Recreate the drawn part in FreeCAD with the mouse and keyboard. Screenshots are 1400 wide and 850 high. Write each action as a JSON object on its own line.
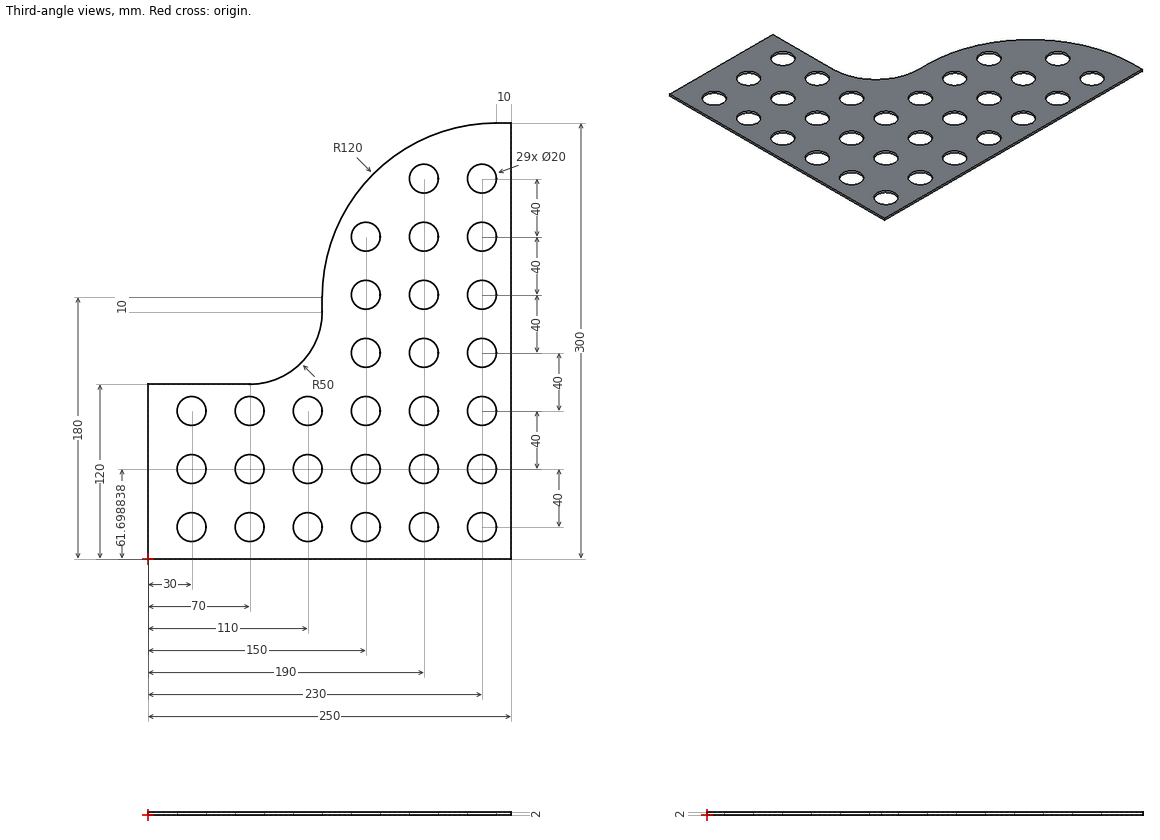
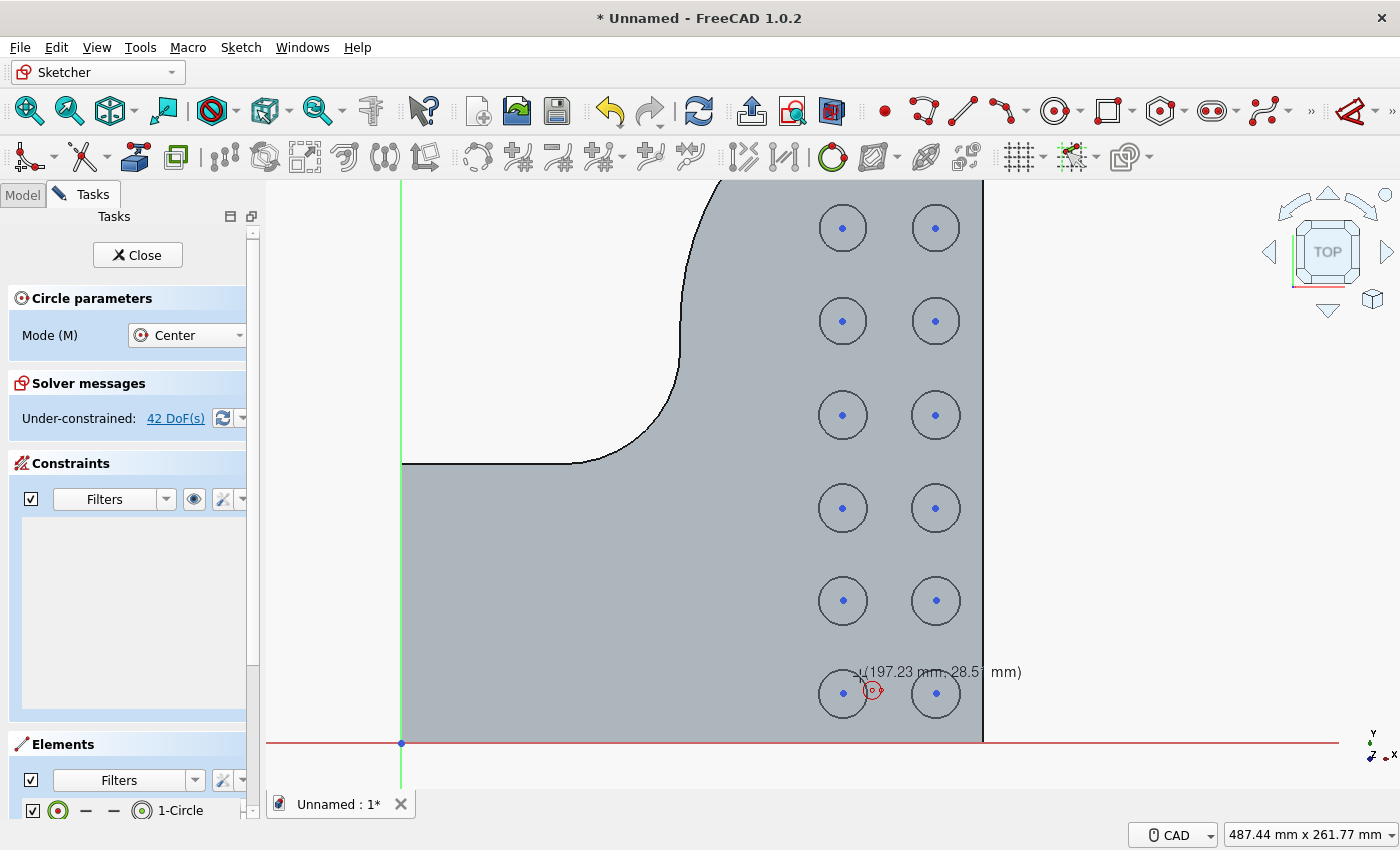
{"action": "left_click", "coordinate": [750, 228]}
{"action": "left_click", "coordinate": [767, 211]}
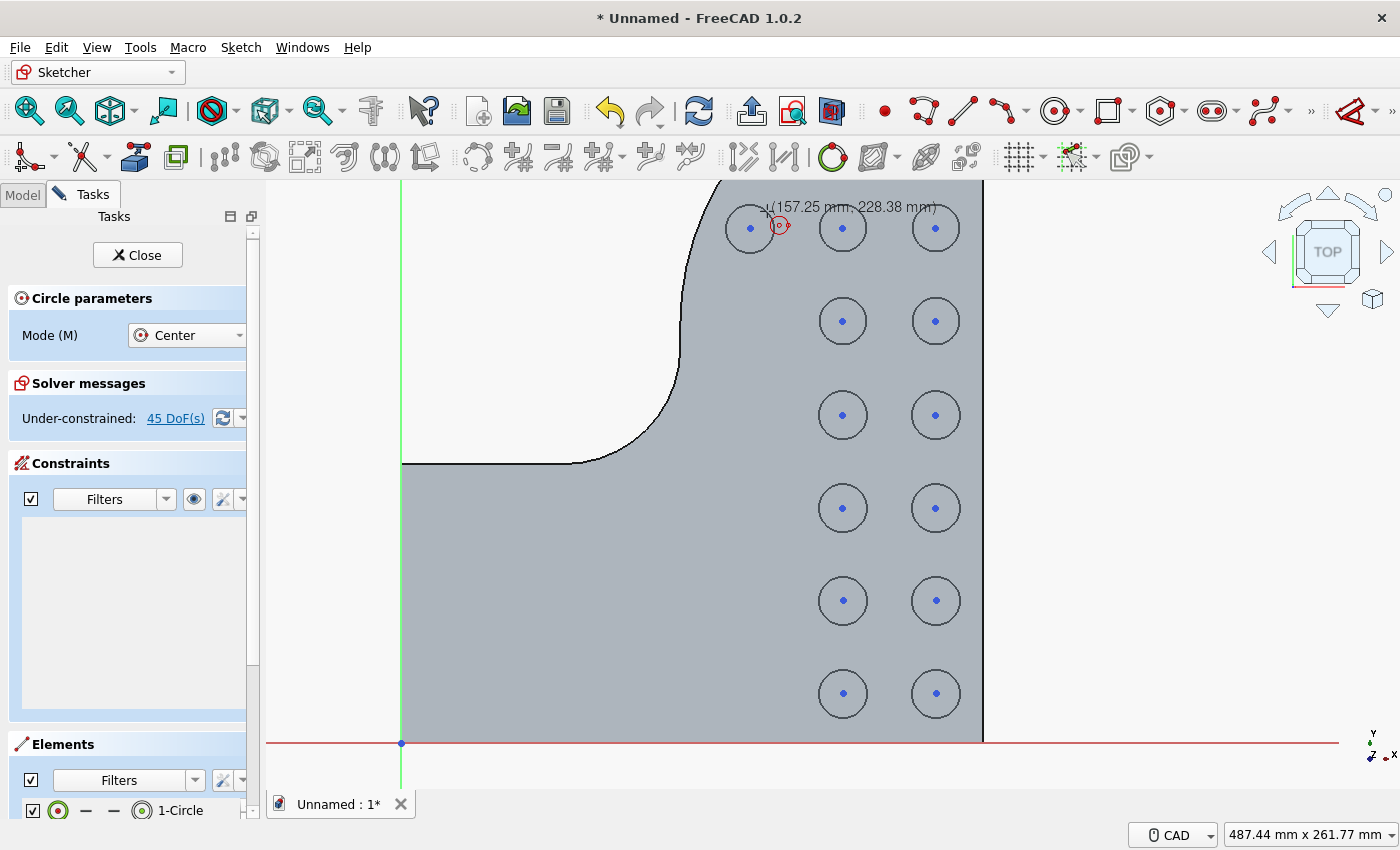
{"action": "left_click", "coordinate": [750, 321]}
{"action": "left_click", "coordinate": [767, 304]}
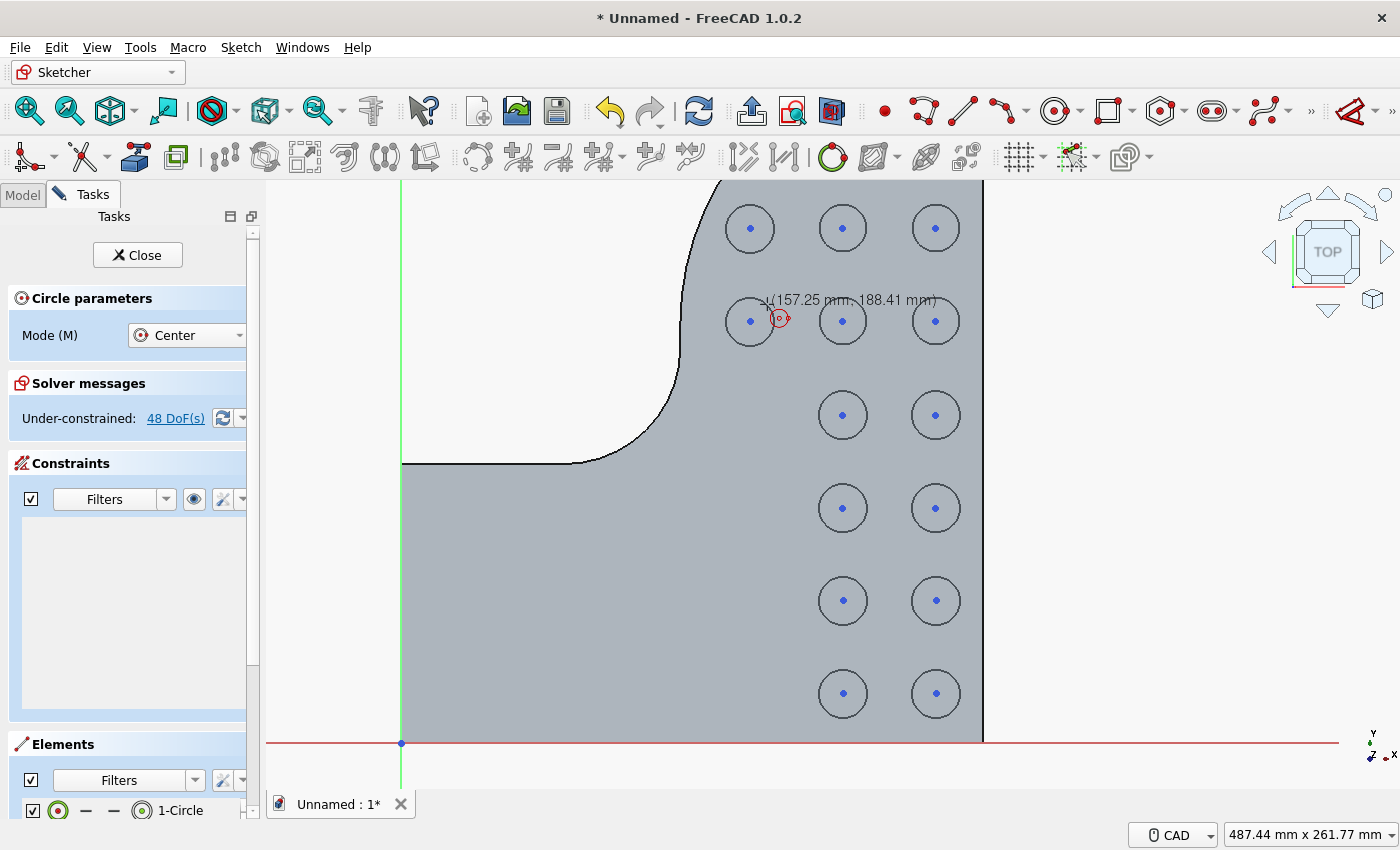
{"action": "left_click", "coordinate": [750, 414]}
{"action": "left_click", "coordinate": [767, 397]}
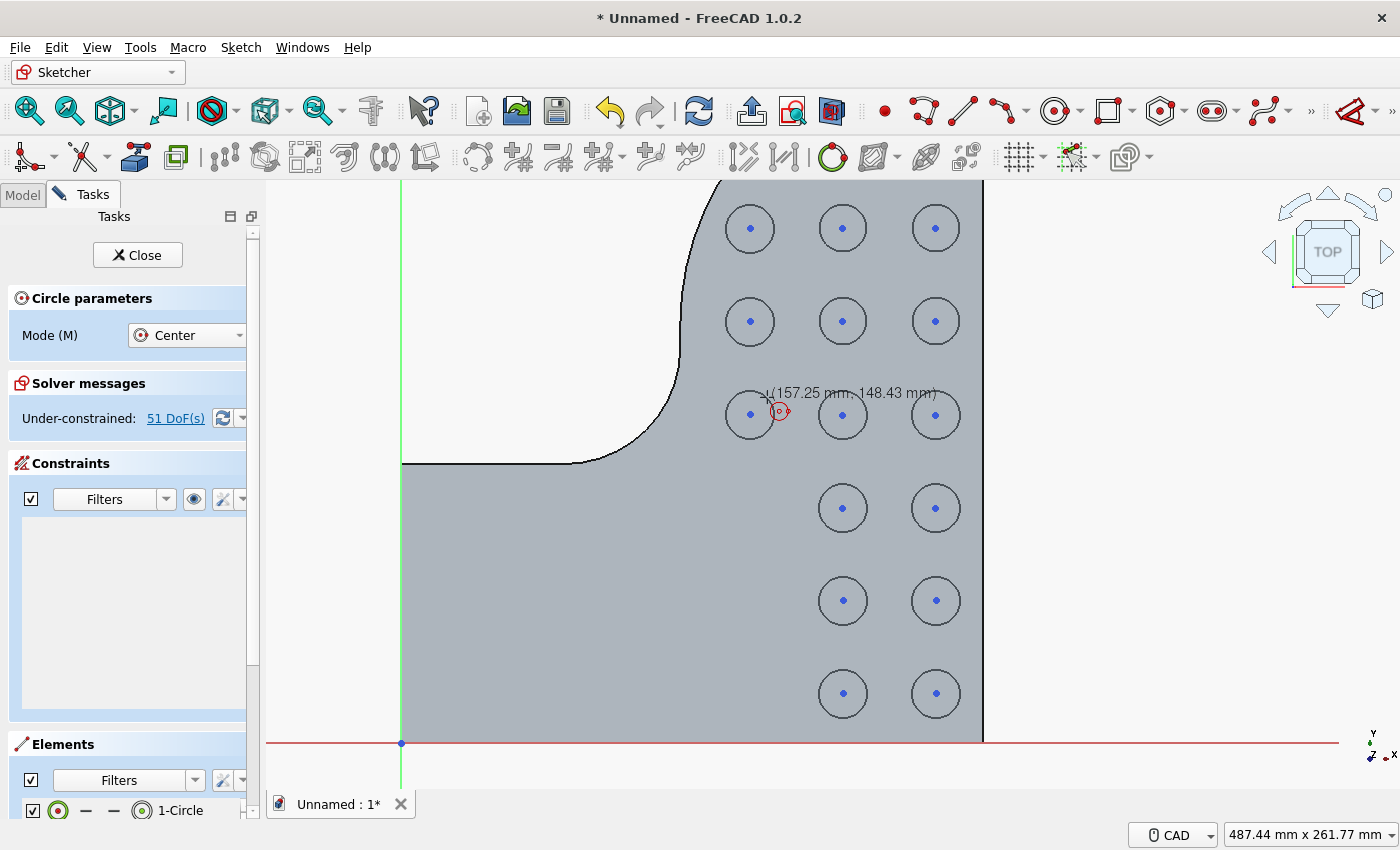
{"action": "left_click", "coordinate": [750, 507]}
{"action": "left_click", "coordinate": [767, 490]}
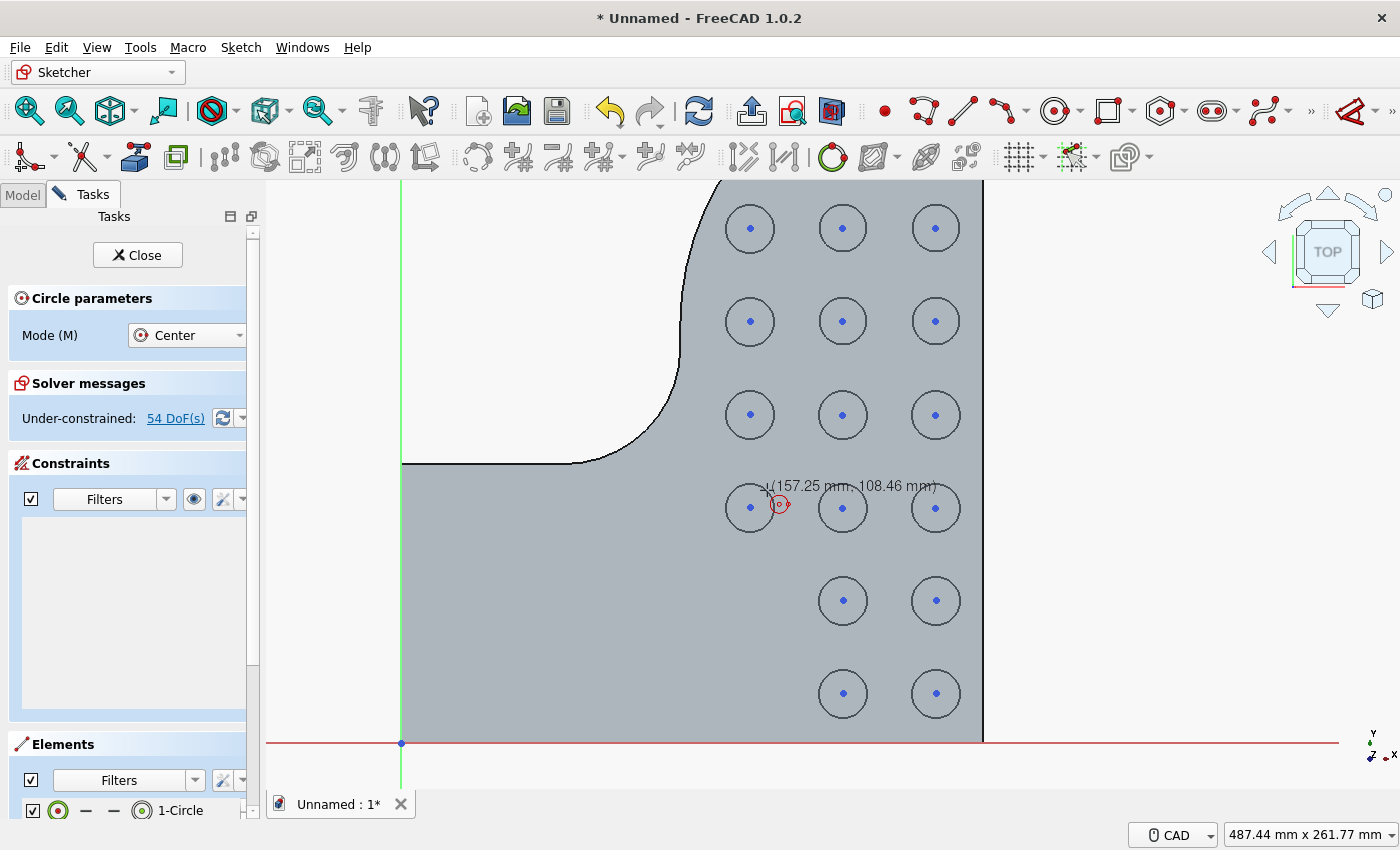
{"action": "left_click", "coordinate": [750, 600]}
{"action": "left_click", "coordinate": [767, 583]}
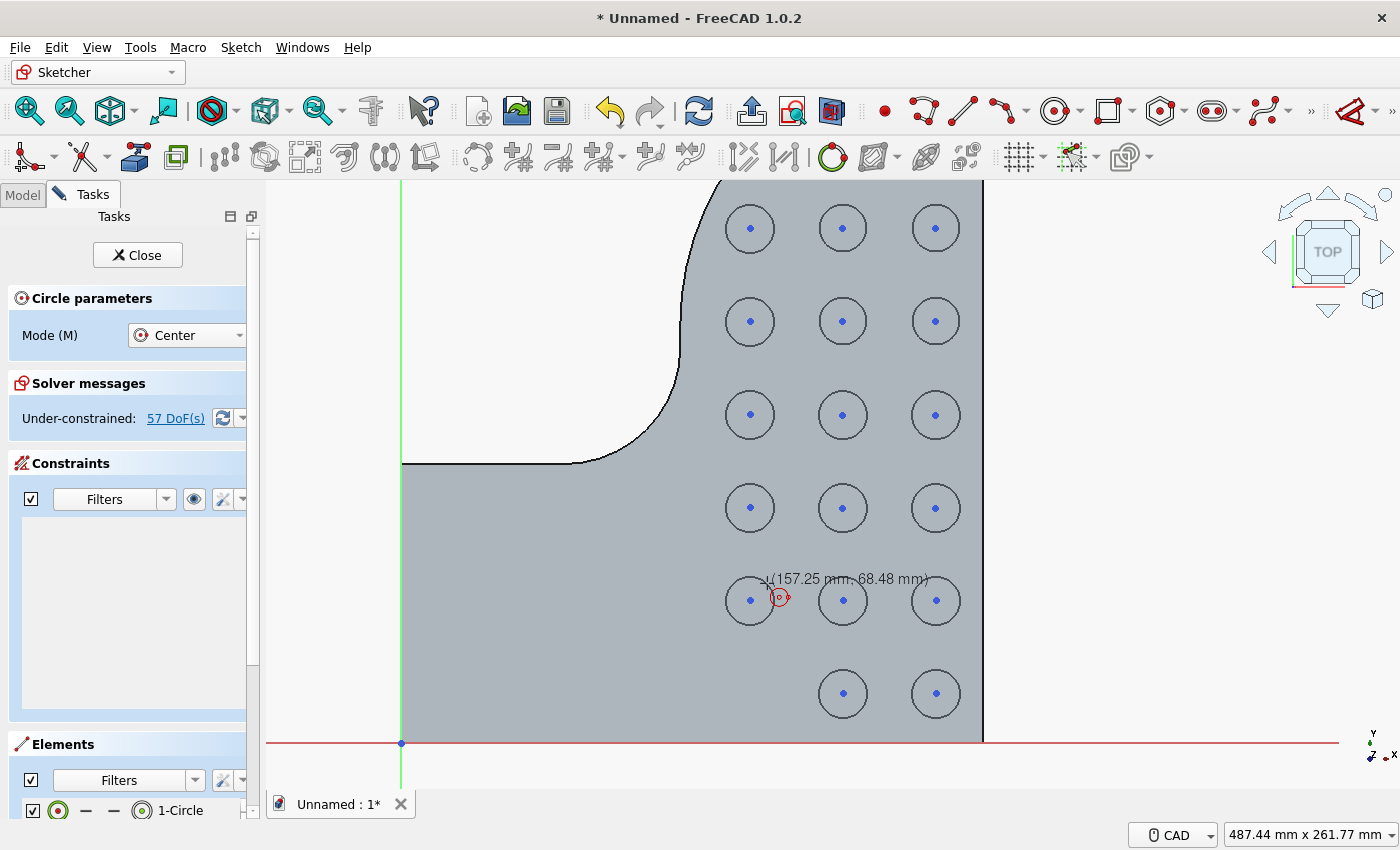
{"action": "left_click", "coordinate": [750, 693]}
{"action": "left_click", "coordinate": [767, 676]}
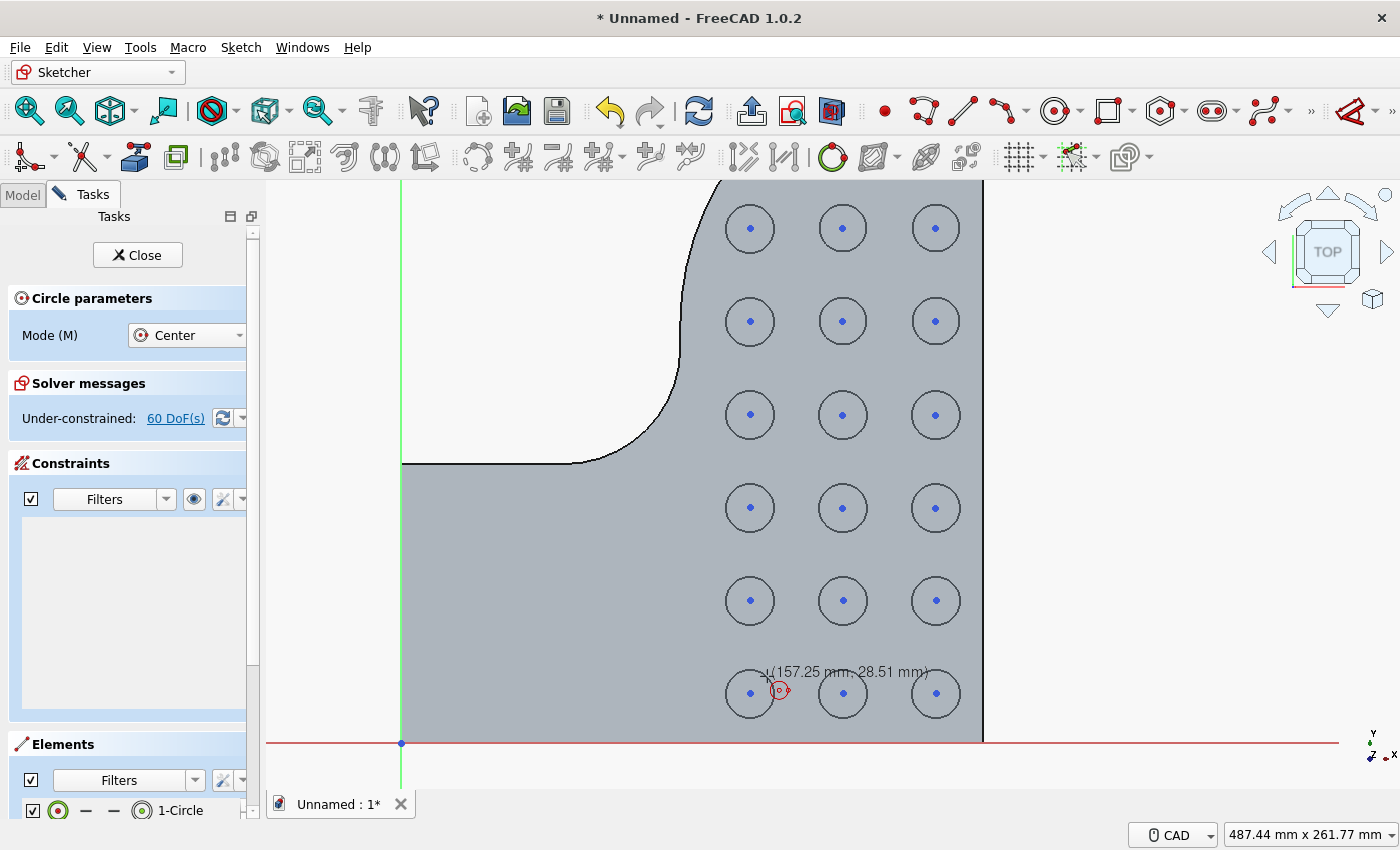
{"action": "left_click", "coordinate": [657, 507]}
{"action": "left_click", "coordinate": [674, 490]}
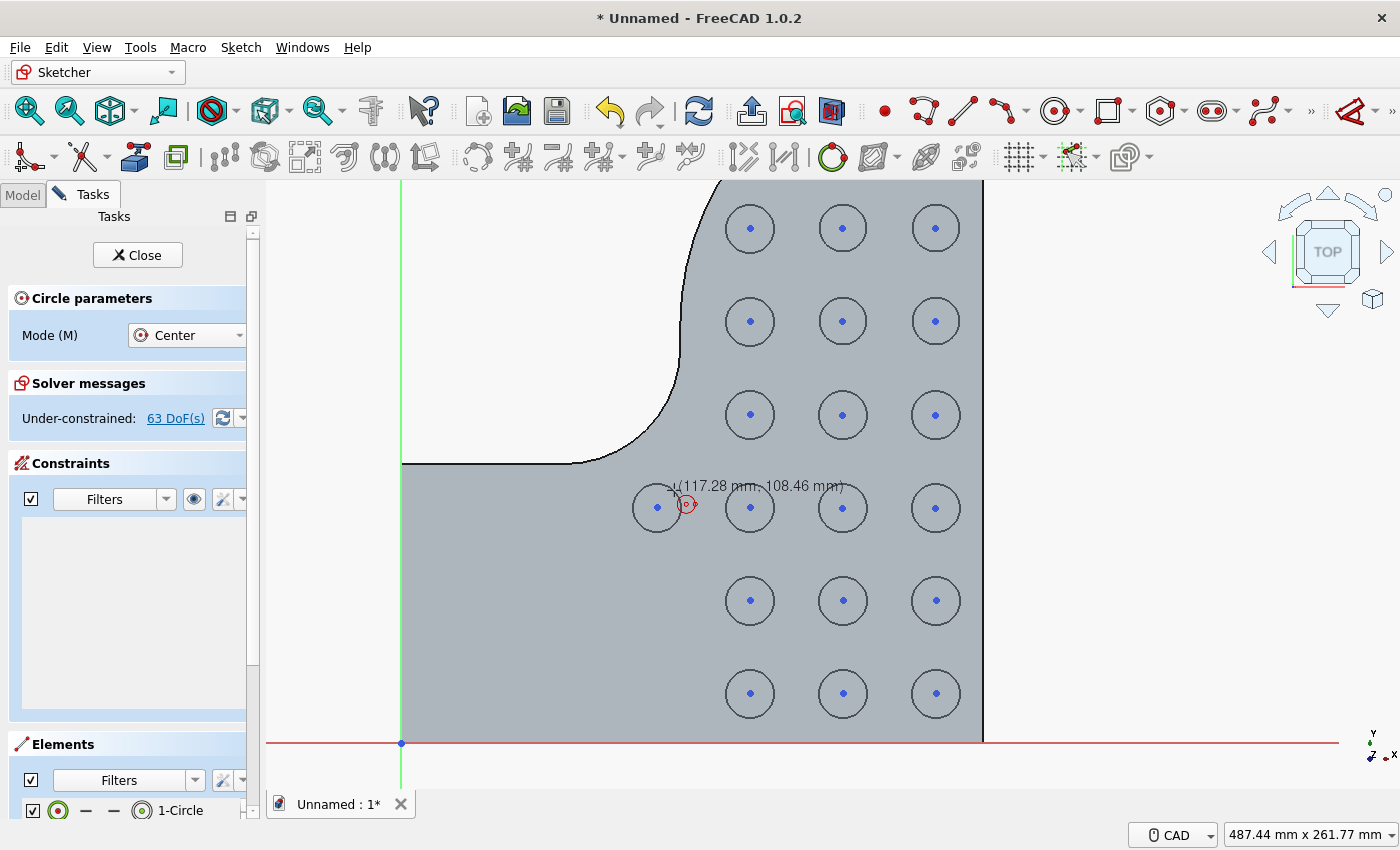
{"action": "left_click", "coordinate": [564, 507]}
{"action": "left_click", "coordinate": [580, 490]}